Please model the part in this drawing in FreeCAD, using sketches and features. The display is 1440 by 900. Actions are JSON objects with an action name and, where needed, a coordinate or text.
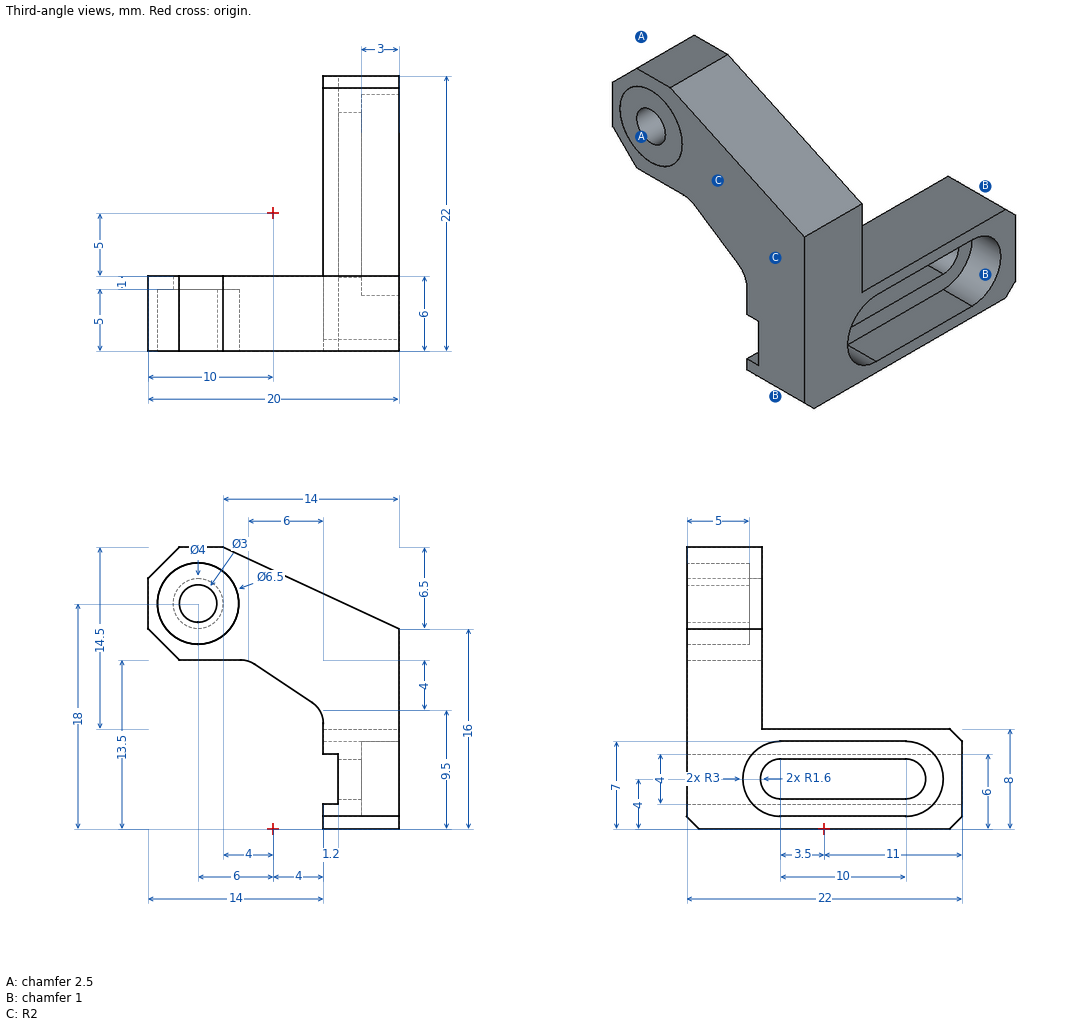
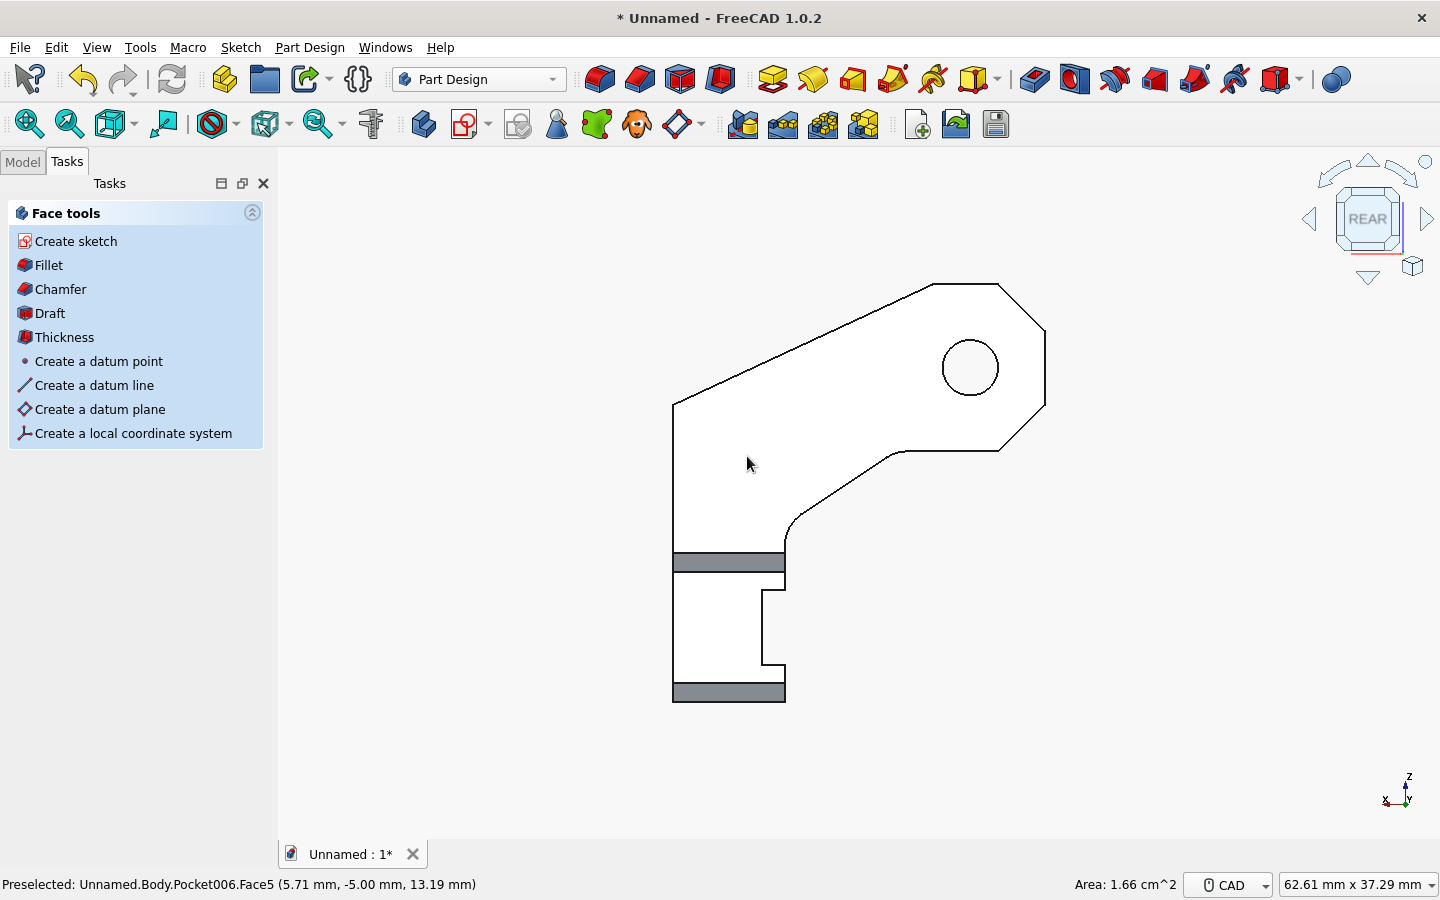
{"action": "left_click", "coordinate": [464, 124]}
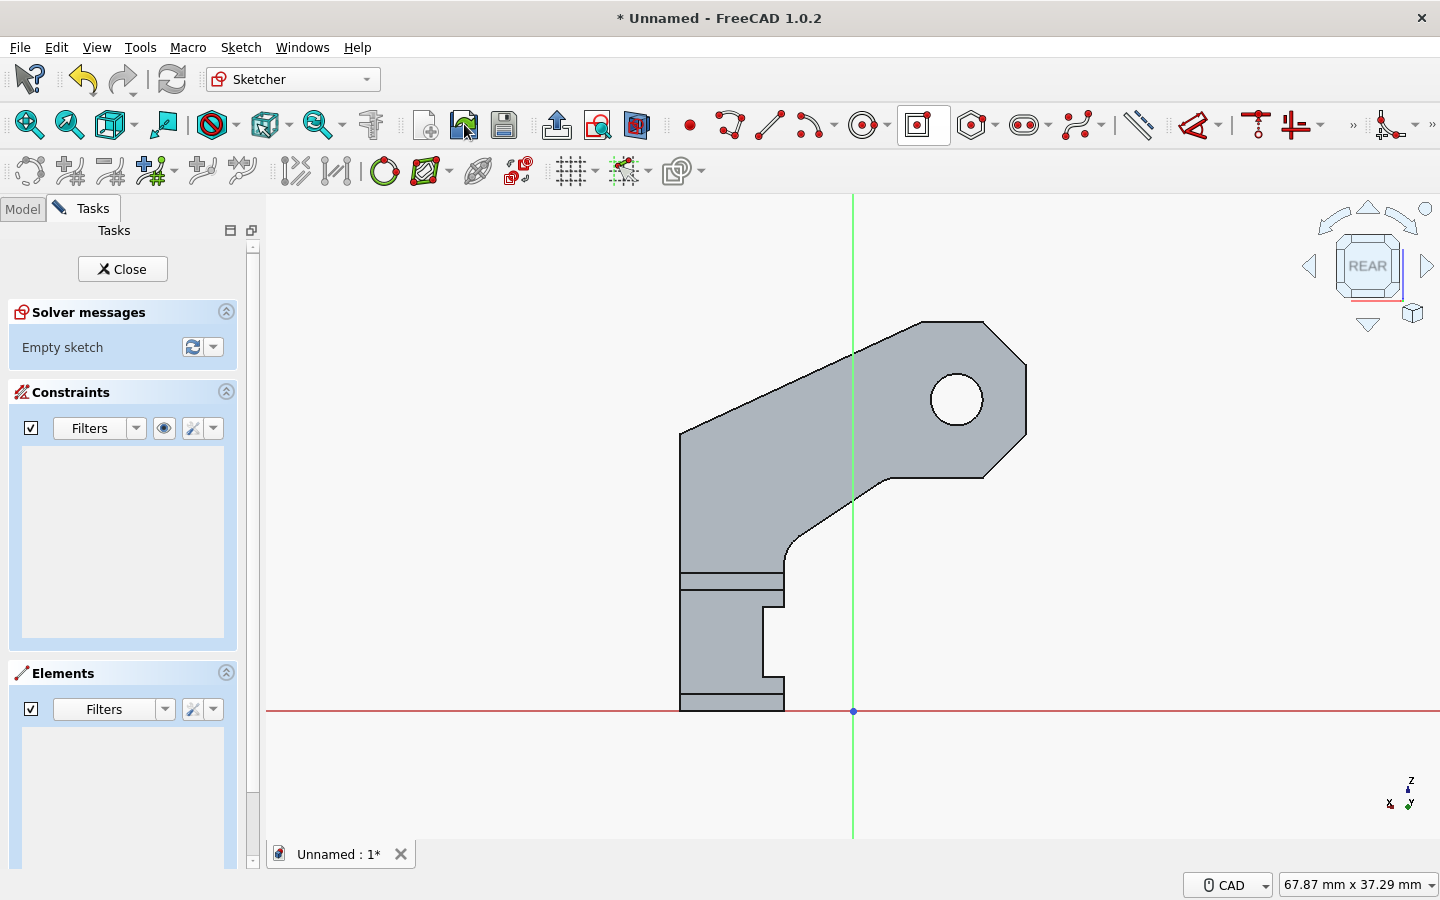
{"action": "left_click", "coordinate": [638, 126]}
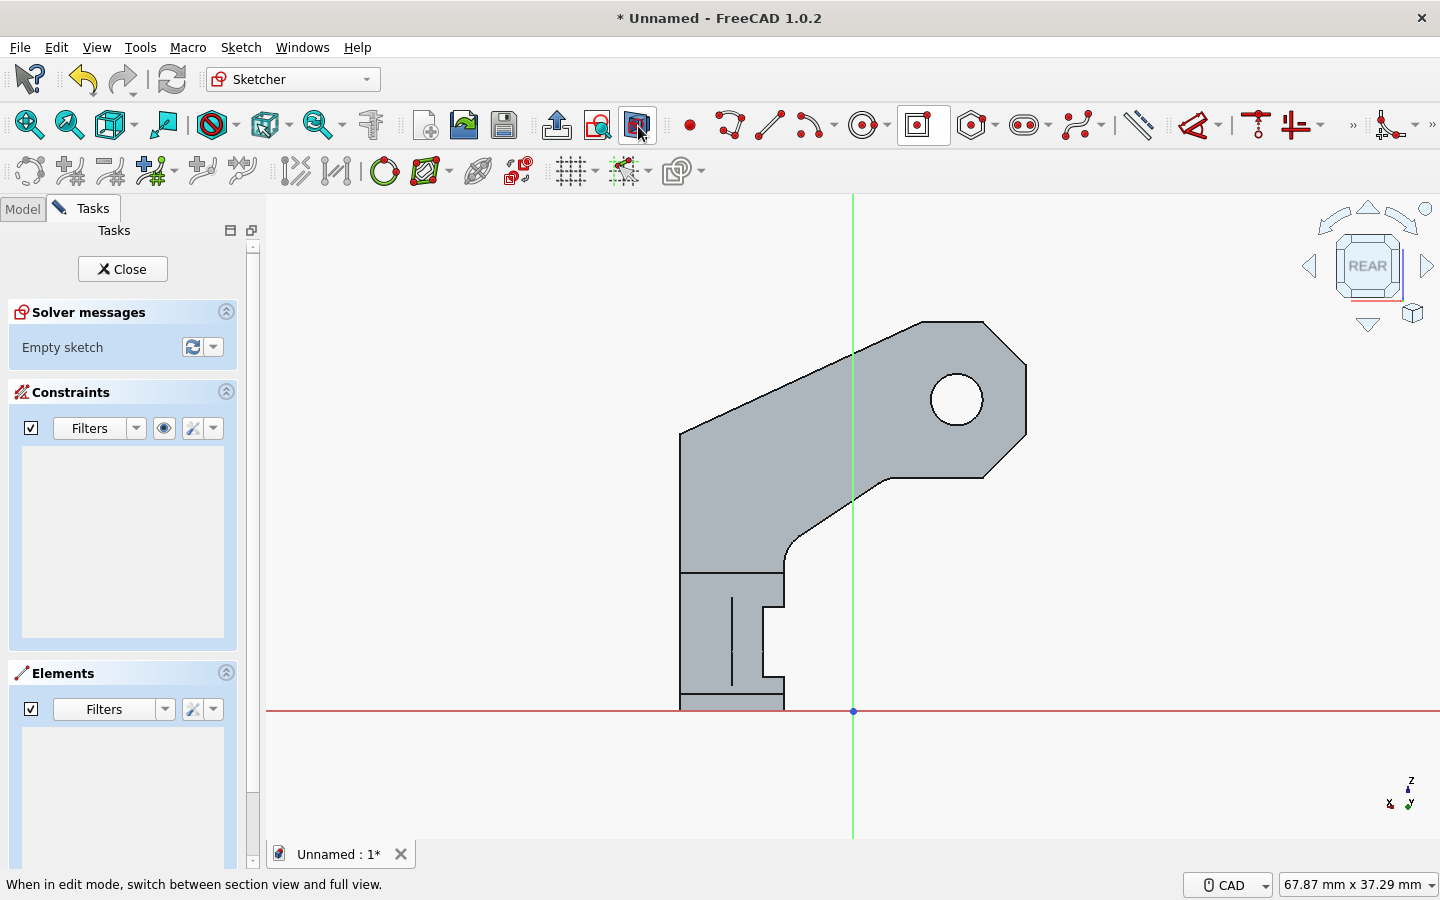
{"action": "scroll", "coordinate": [991, 377], "scroll_direction": "up", "scroll_amount": 9}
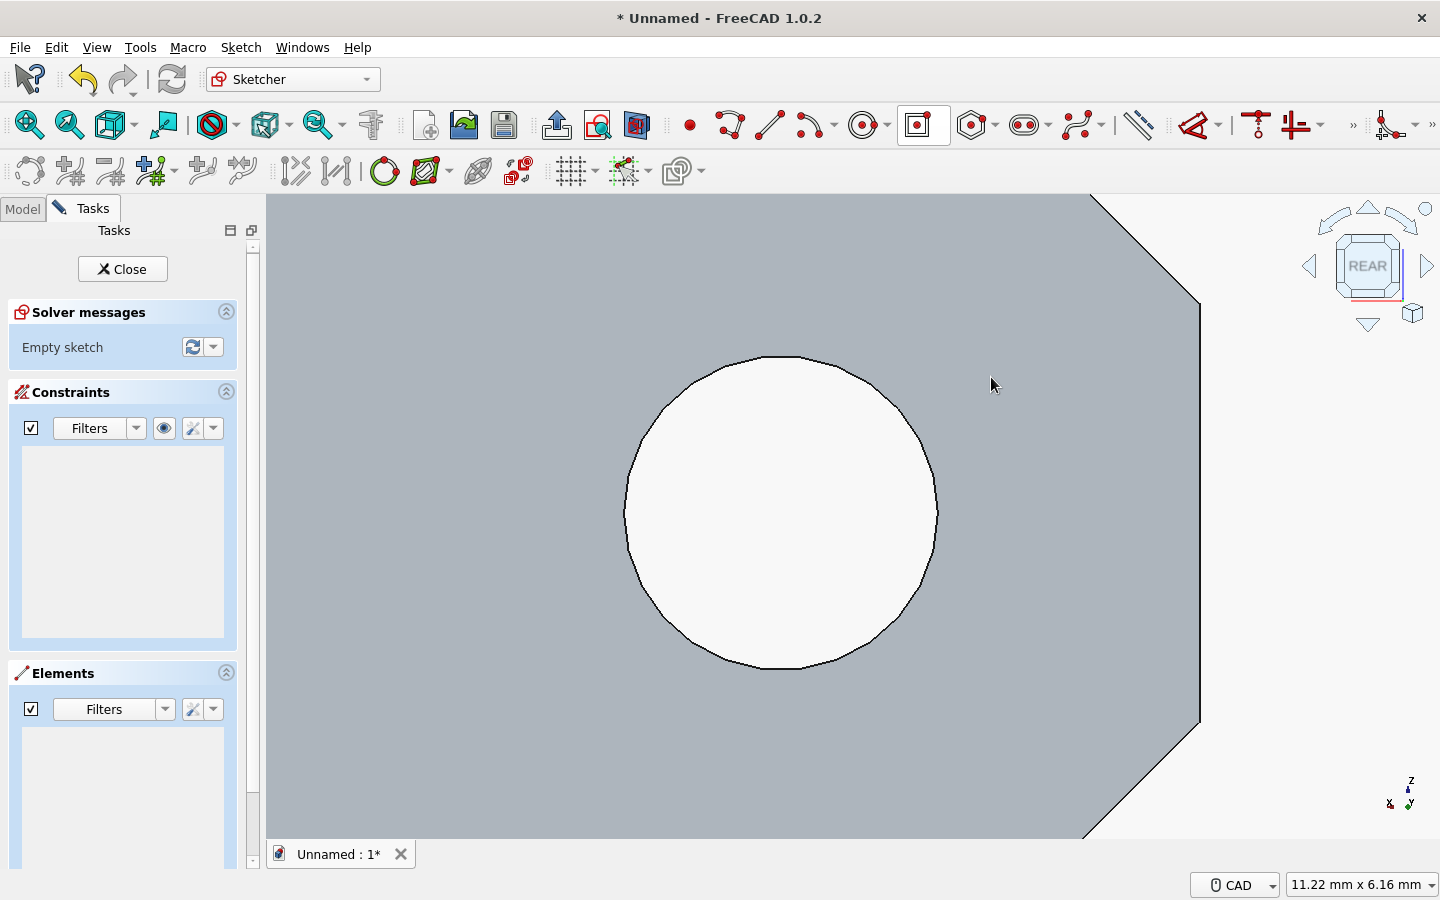
{"action": "left_click", "coordinate": [864, 126]}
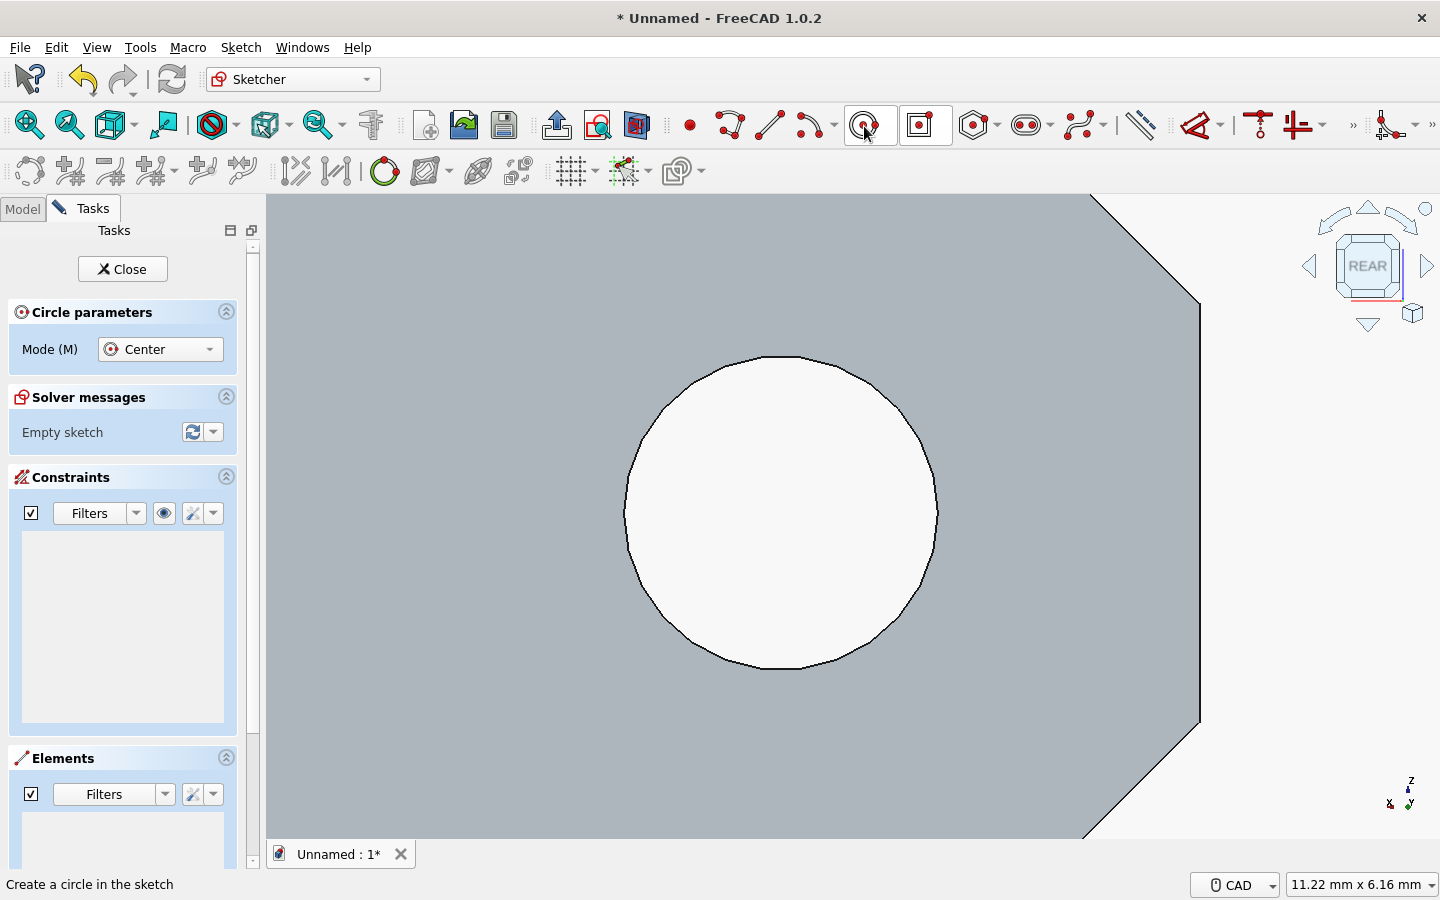
{"action": "left_click", "coordinate": [781, 513]}
{"action": "mouse_move", "coordinate": [929, 365]}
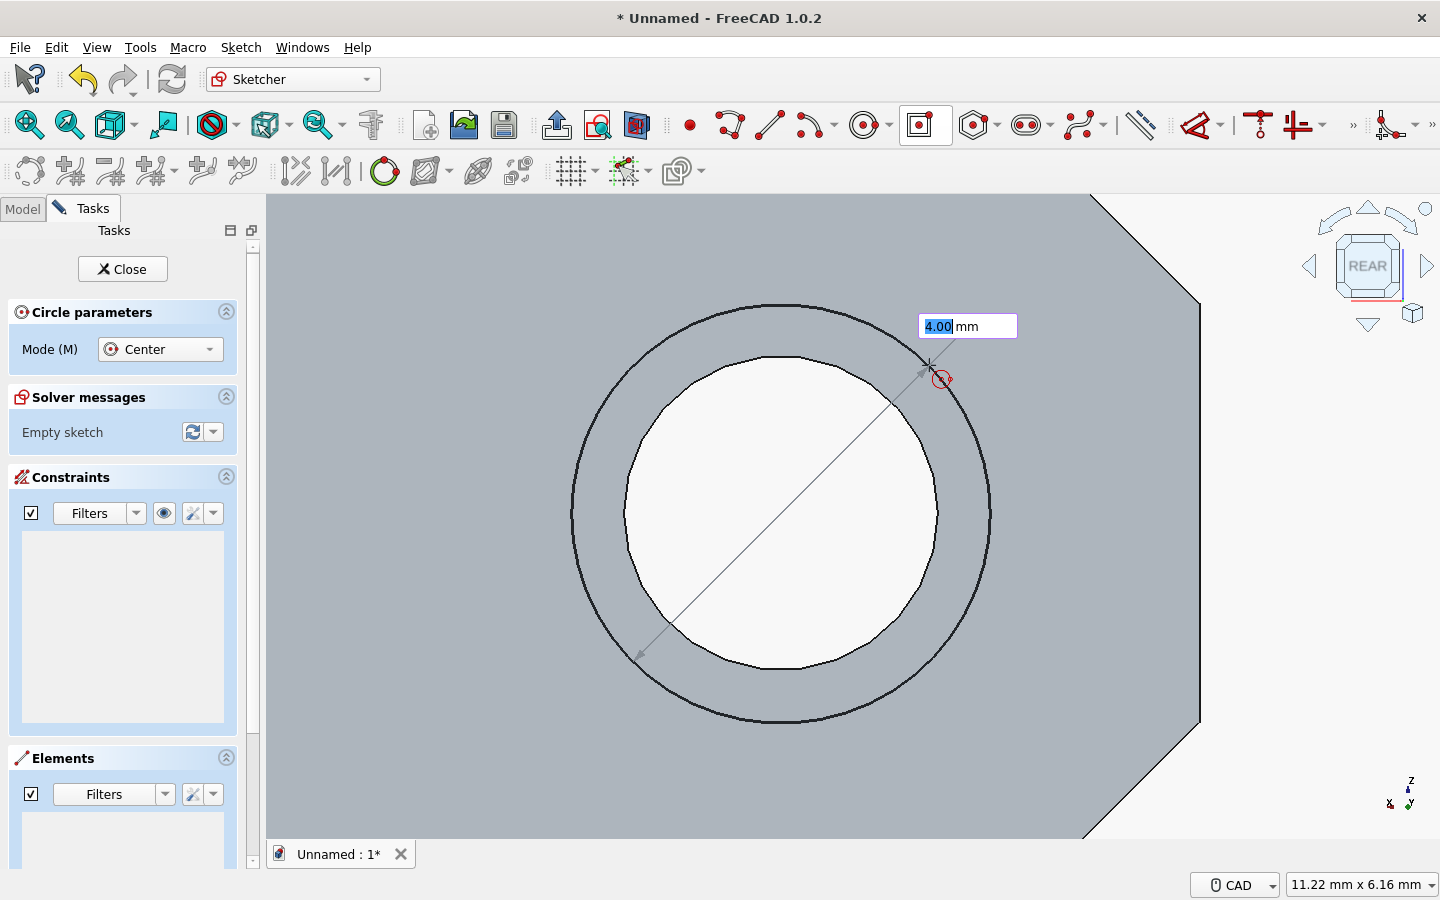
{"action": "type", "text": "4"}
{"action": "key", "text": "Return"}
{"action": "key", "text": "Escape"}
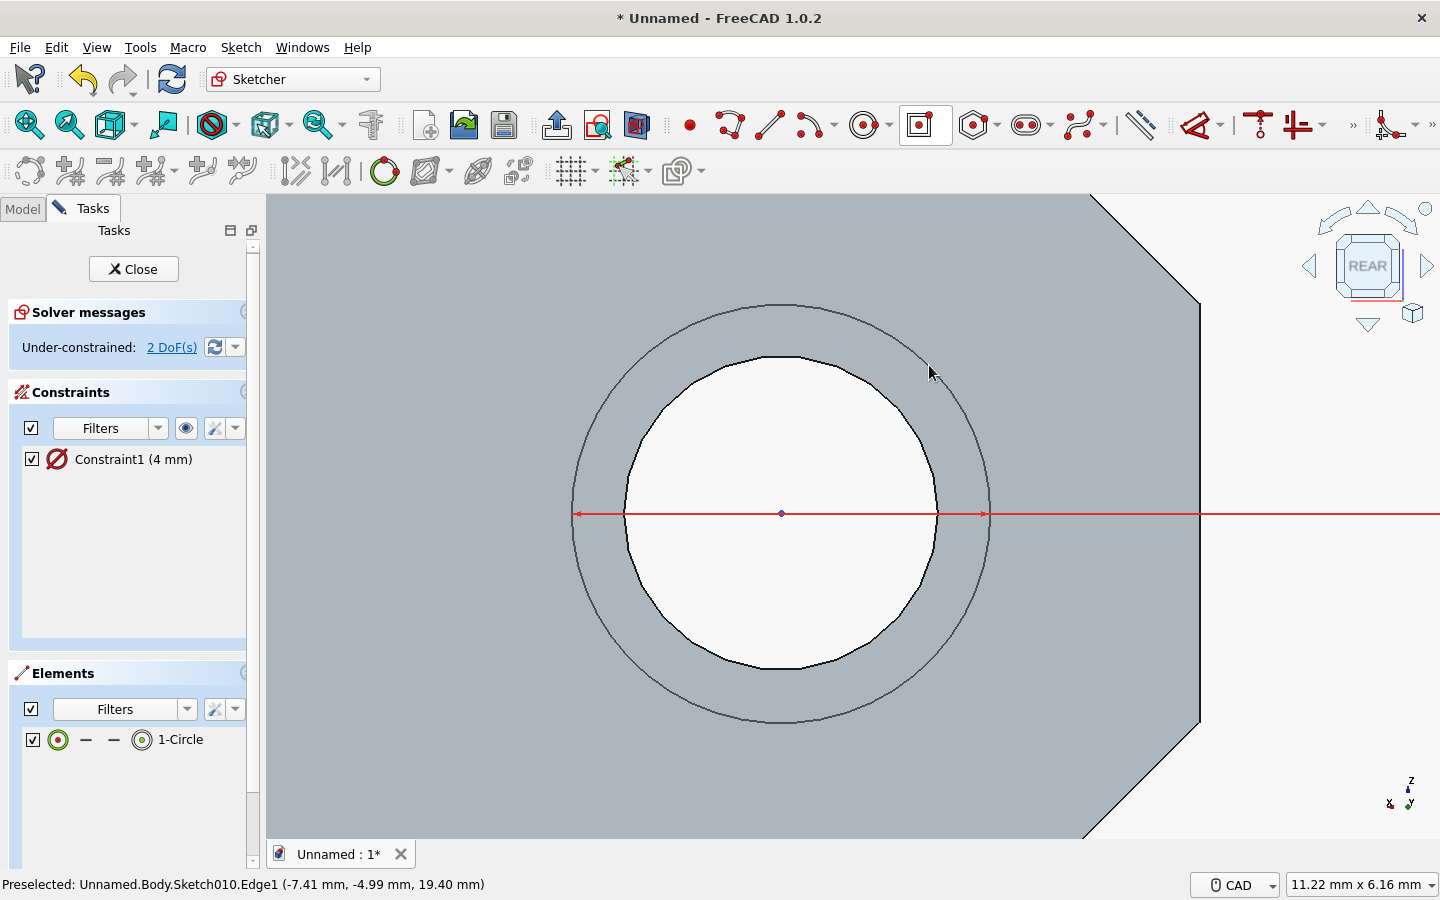
{"action": "left_click", "coordinate": [1196, 126]}